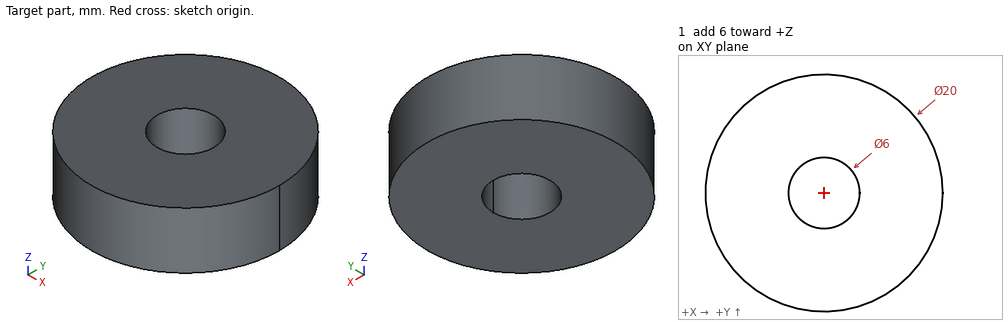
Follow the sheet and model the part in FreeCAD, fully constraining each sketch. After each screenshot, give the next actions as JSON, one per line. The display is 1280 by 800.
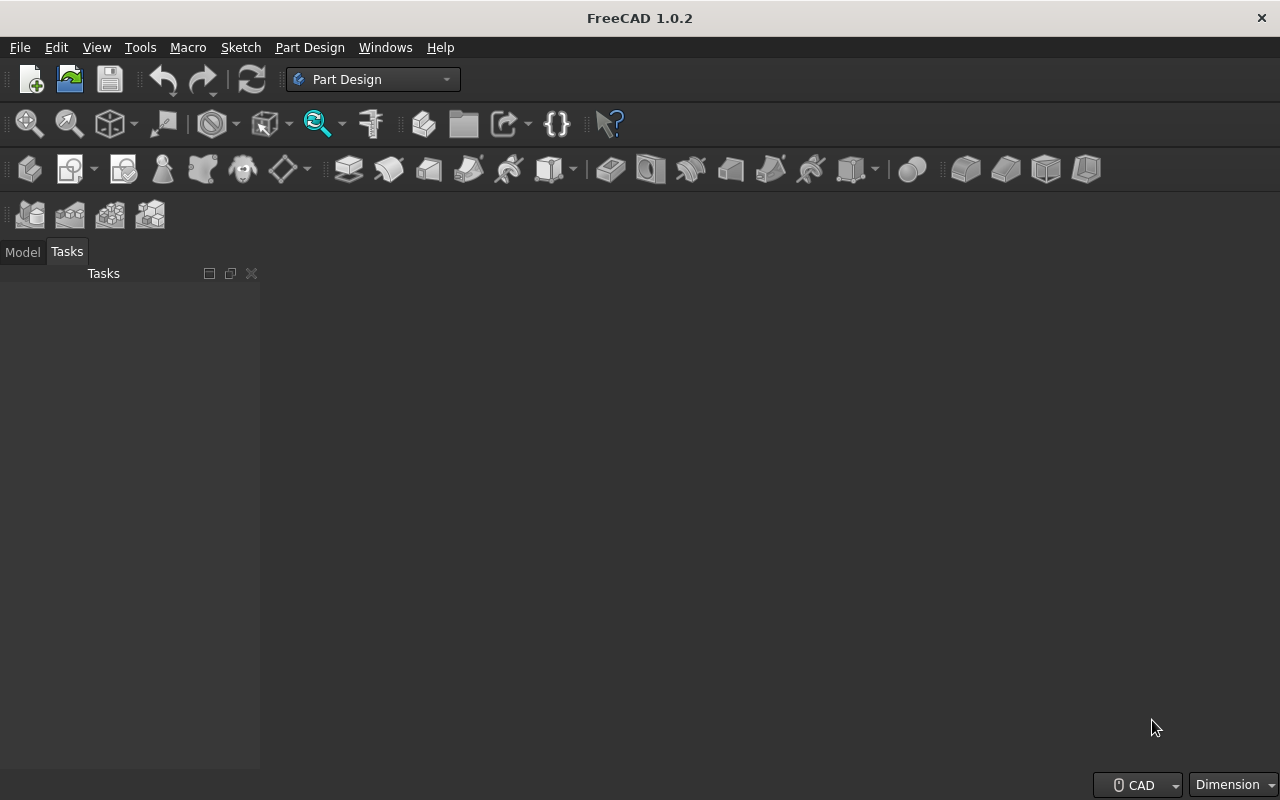
{"action": "left_click", "coordinate": [30, 80]}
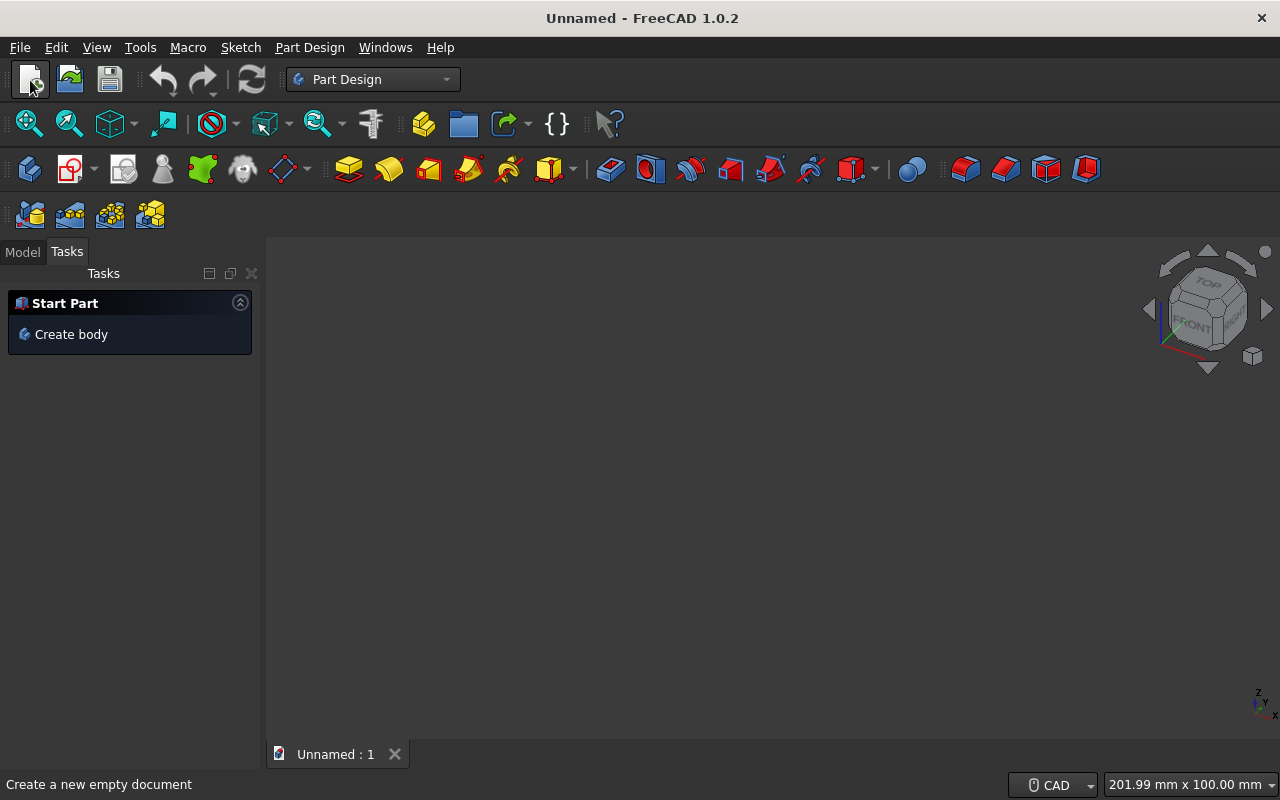
{"action": "left_click", "coordinate": [70, 170]}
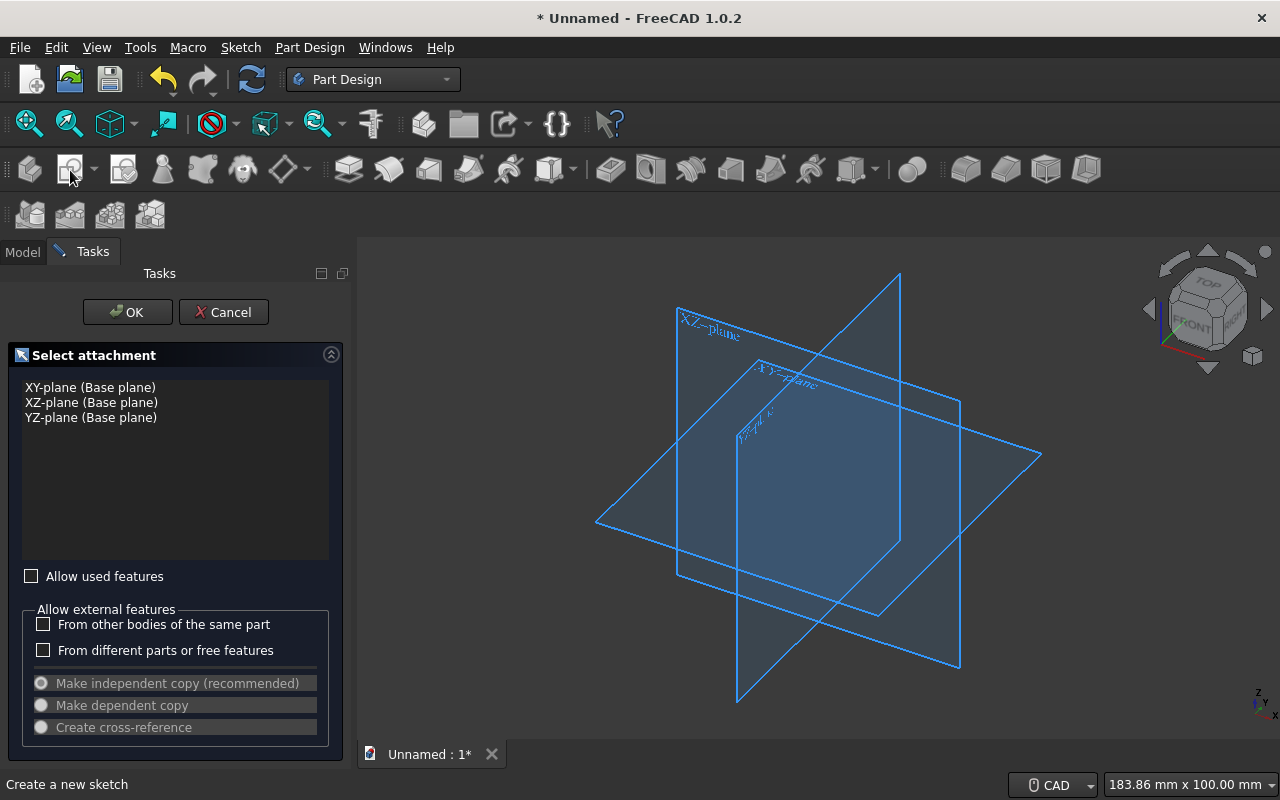
{"action": "left_click", "coordinate": [82, 388]}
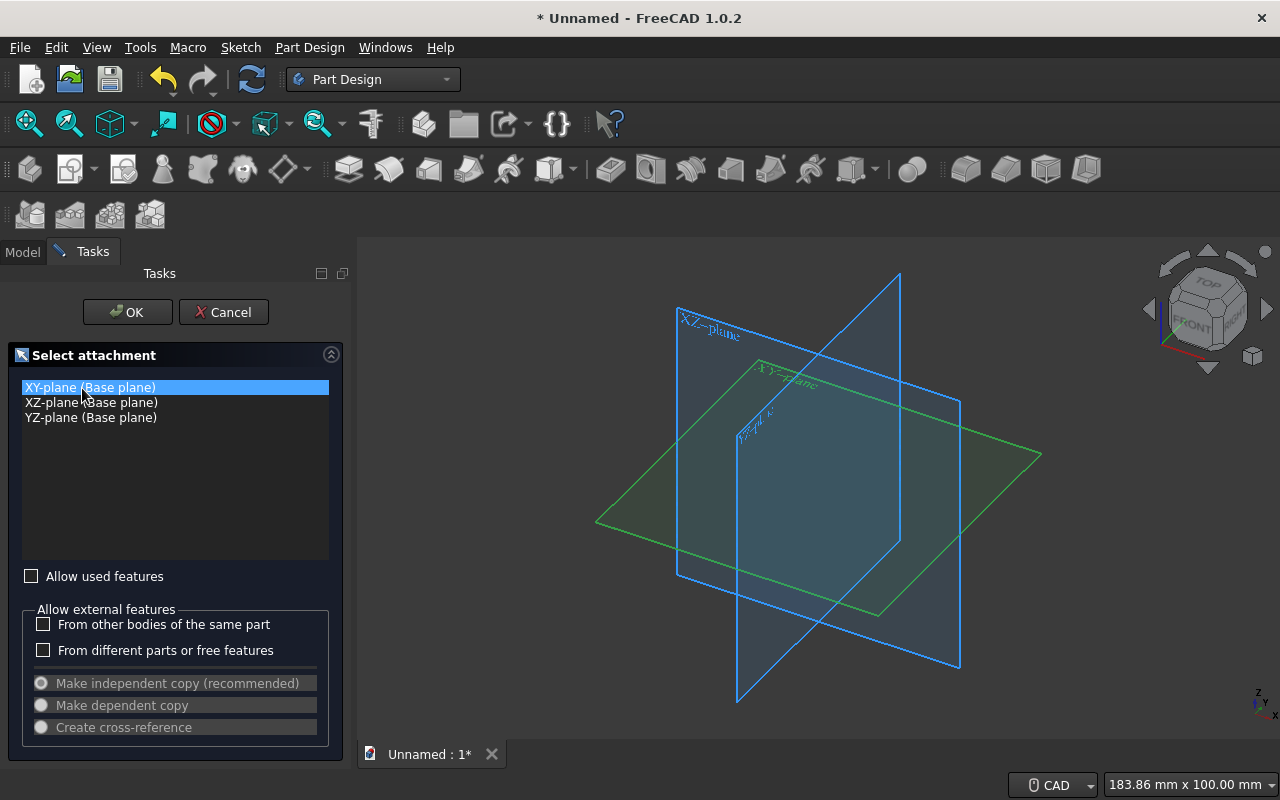
{"action": "left_click", "coordinate": [128, 312]}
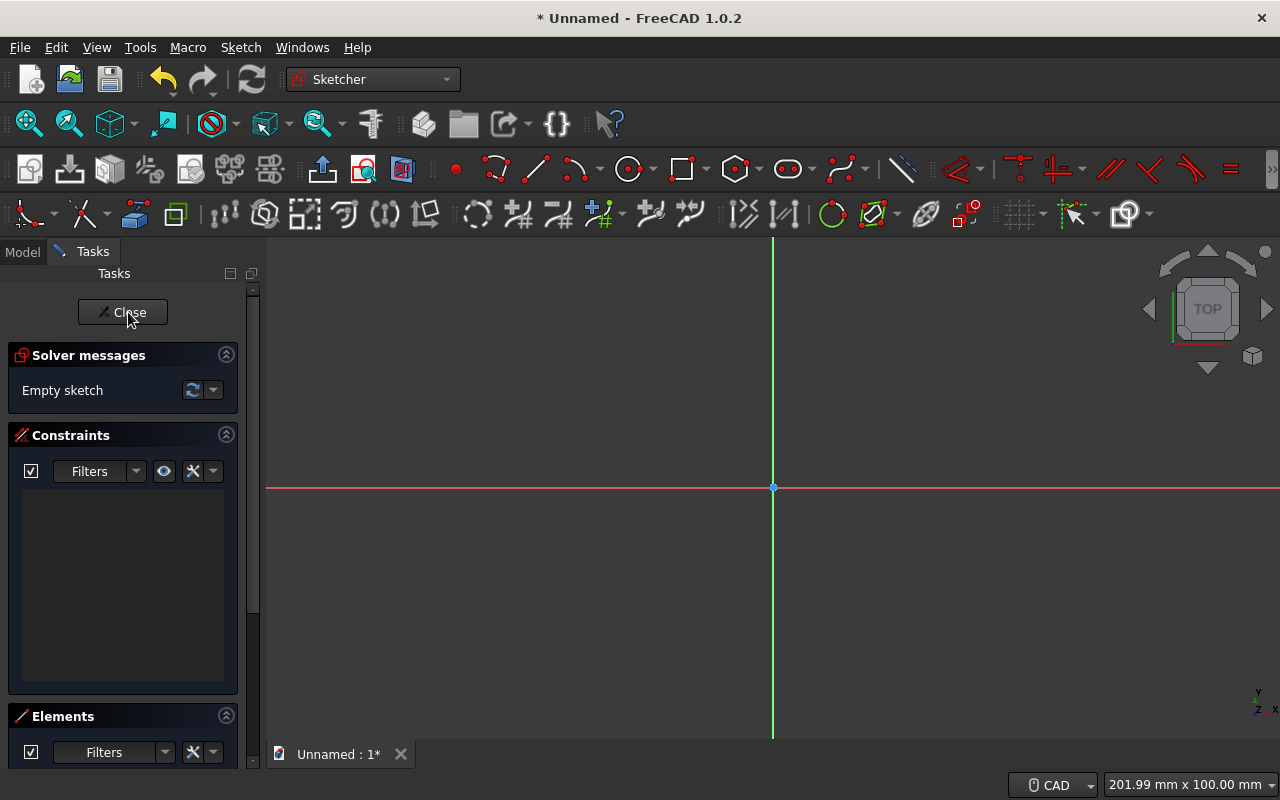
{"action": "scroll", "coordinate": [803, 488], "scroll_direction": "up", "scroll_amount": 6}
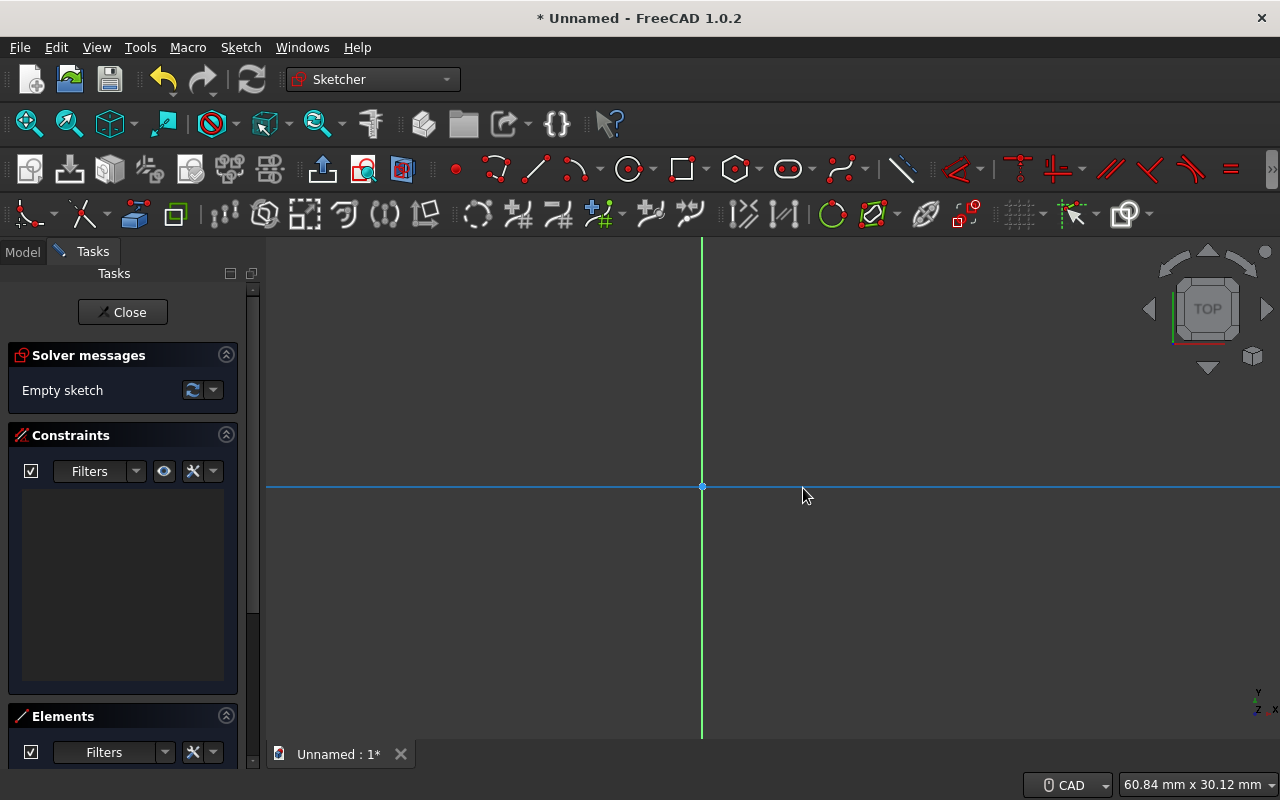
{"action": "left_click", "coordinate": [630, 170]}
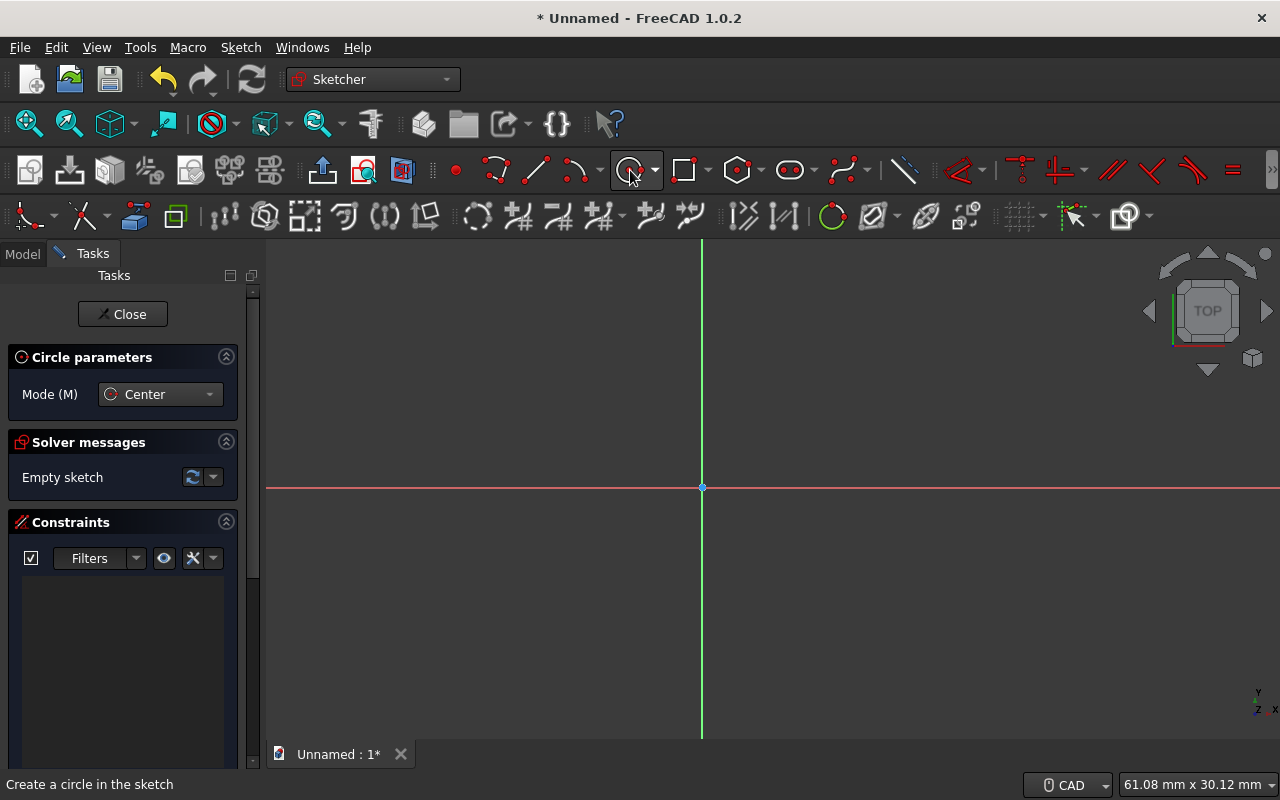
{"action": "left_click", "coordinate": [702, 488]}
{"action": "mouse_move", "coordinate": [820, 370]}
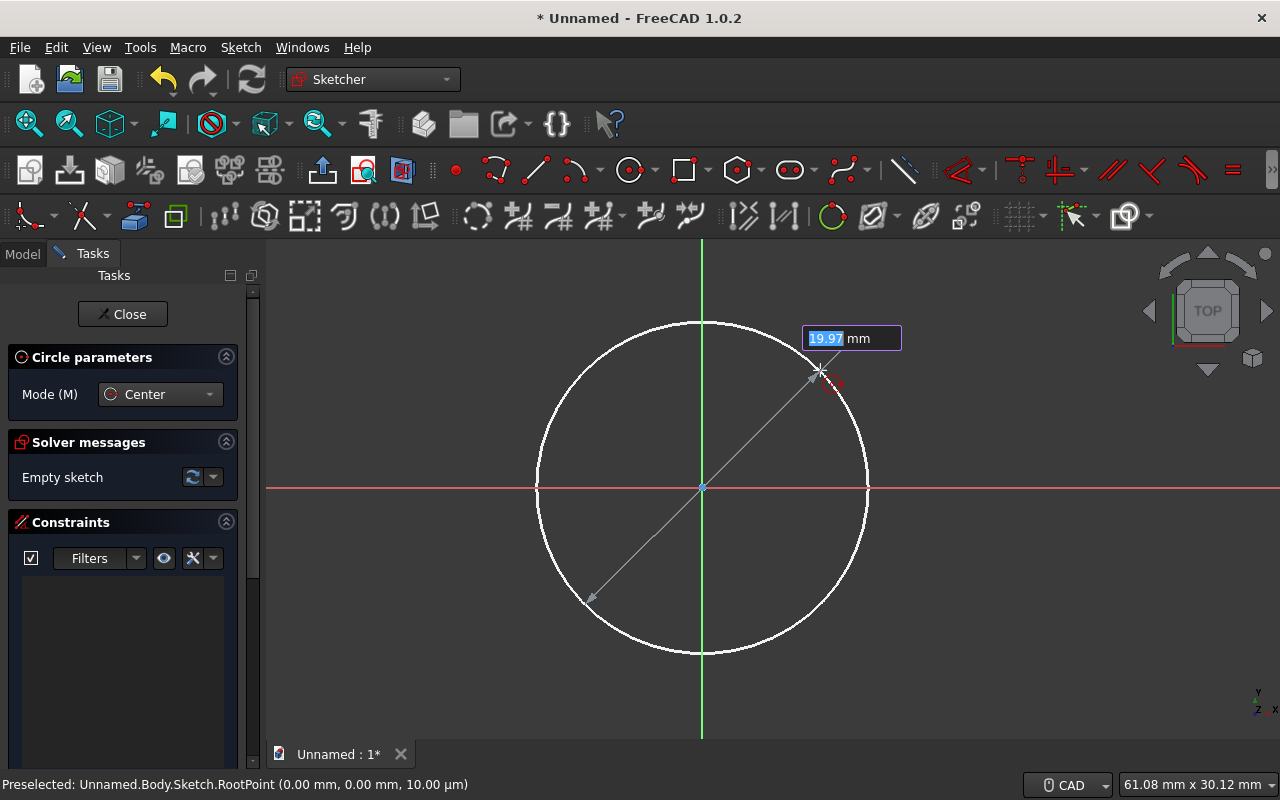
{"action": "type", "text": "20"}
{"action": "key", "text": "Return"}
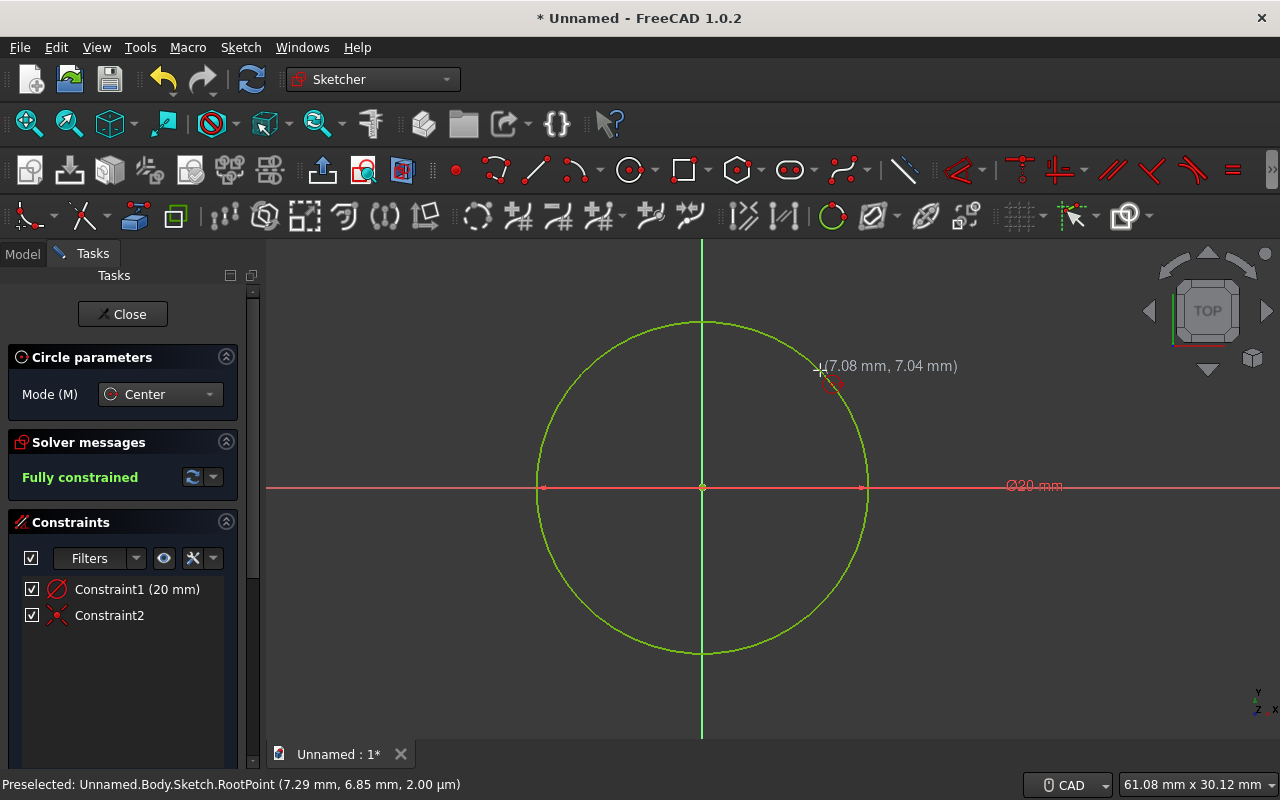
{"action": "left_click", "coordinate": [702, 488]}
{"action": "mouse_move", "coordinate": [738, 453]}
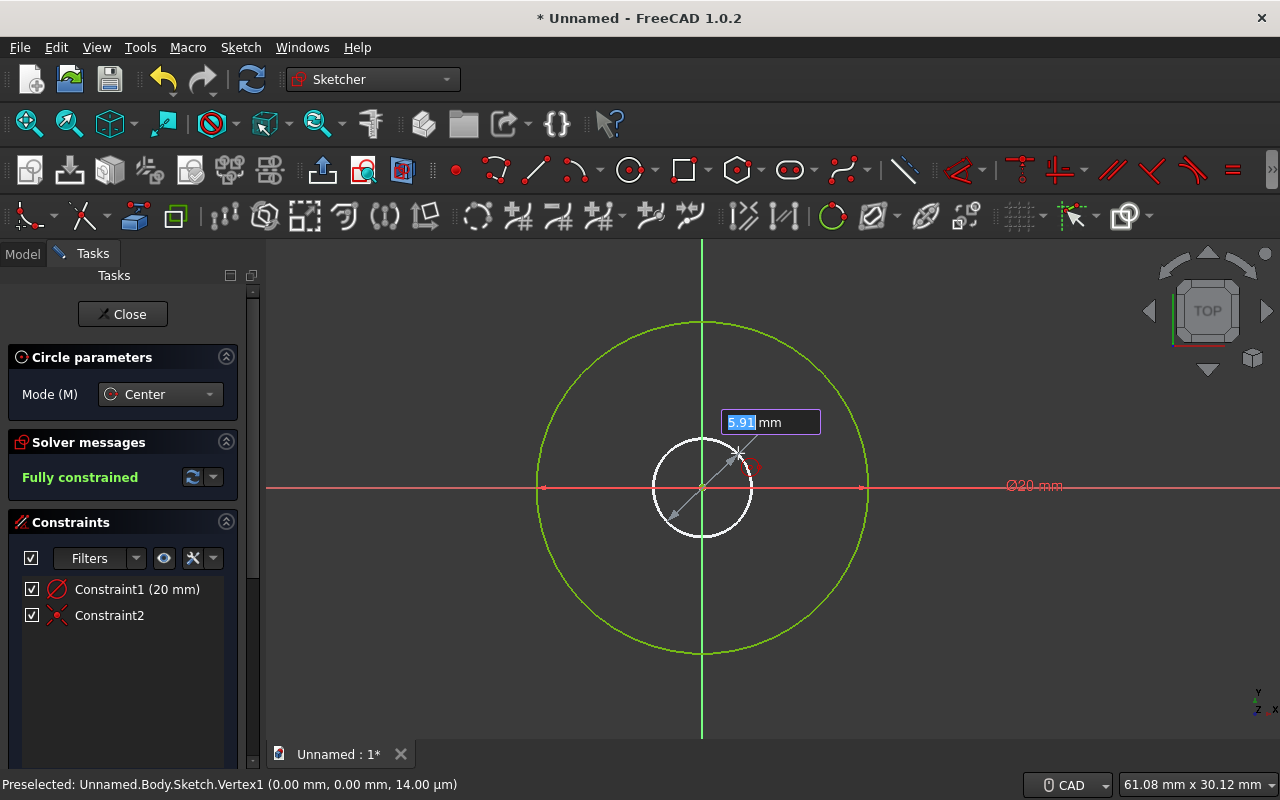
{"action": "type", "text": "6"}
{"action": "key", "text": "Return"}
{"action": "key", "text": "Escape"}